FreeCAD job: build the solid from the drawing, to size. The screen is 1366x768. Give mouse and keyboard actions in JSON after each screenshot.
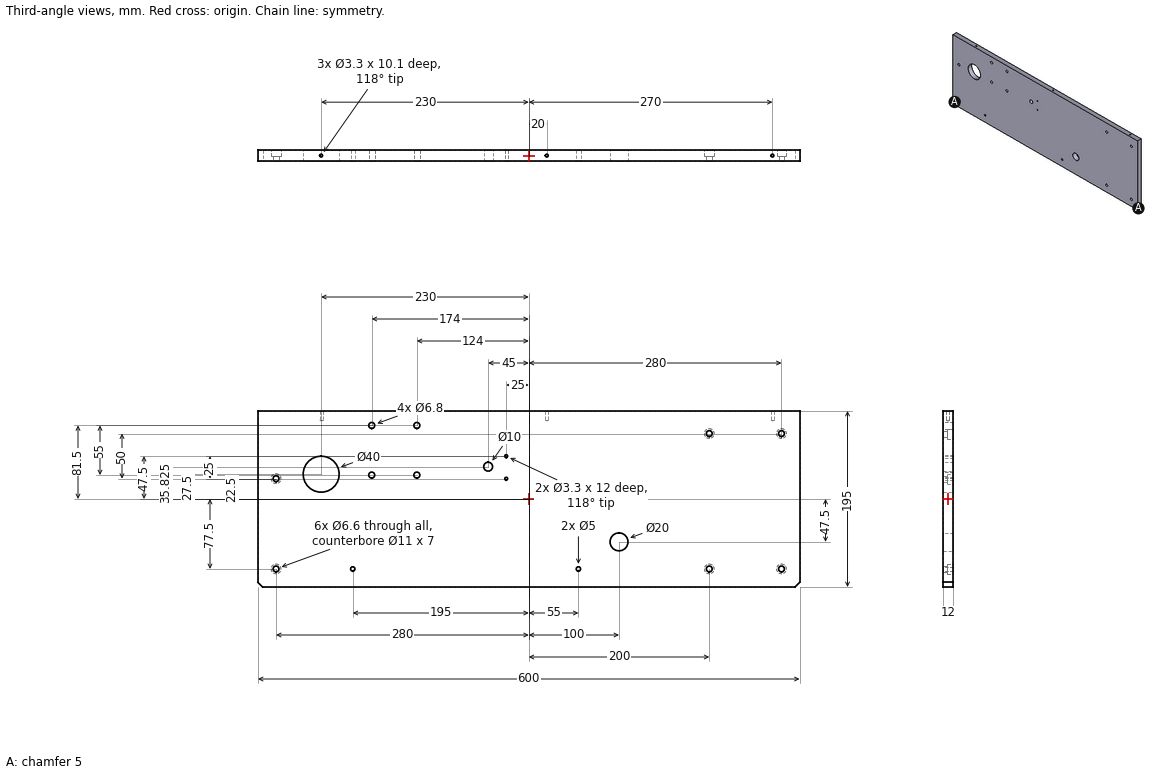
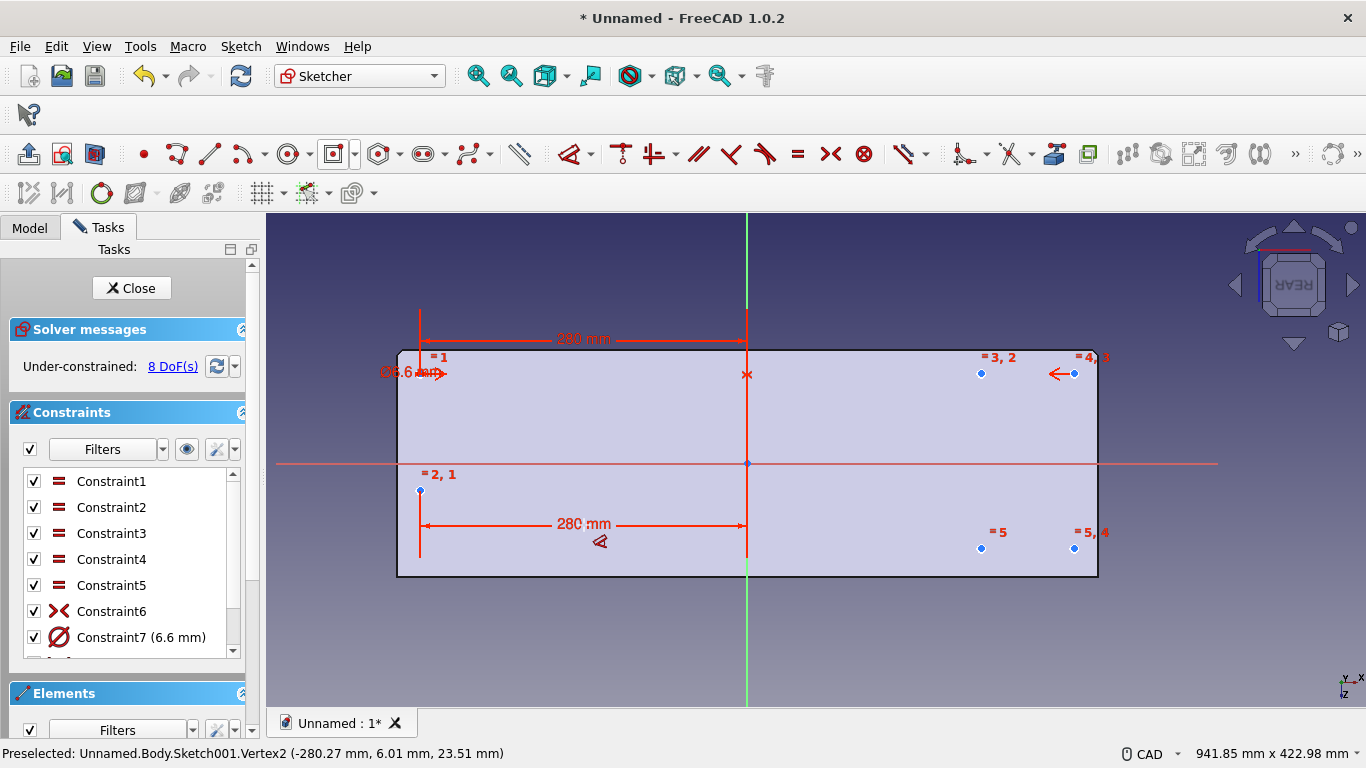
{"action": "left_click", "coordinate": [981, 374]}
{"action": "left_click", "coordinate": [864, 340]}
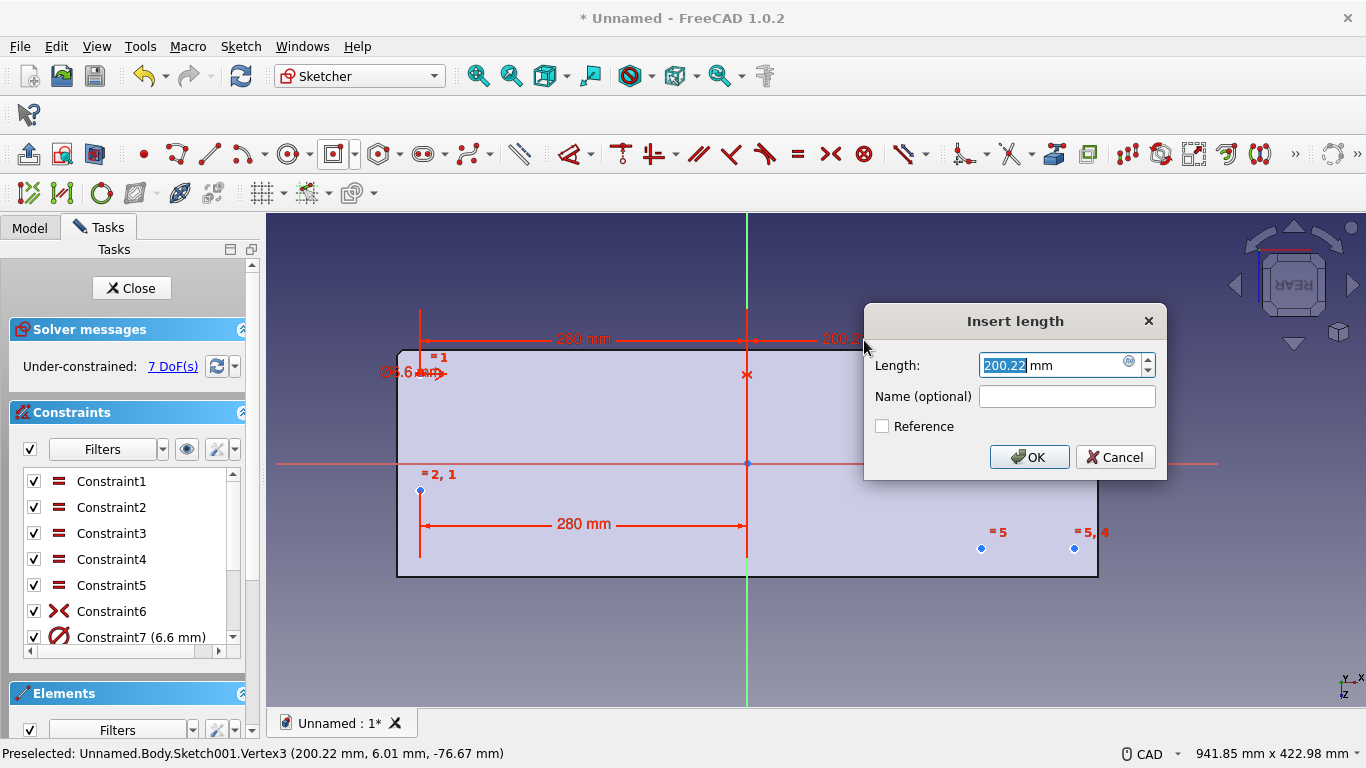
{"action": "type", "text": "200"}
{"action": "key", "text": "Return"}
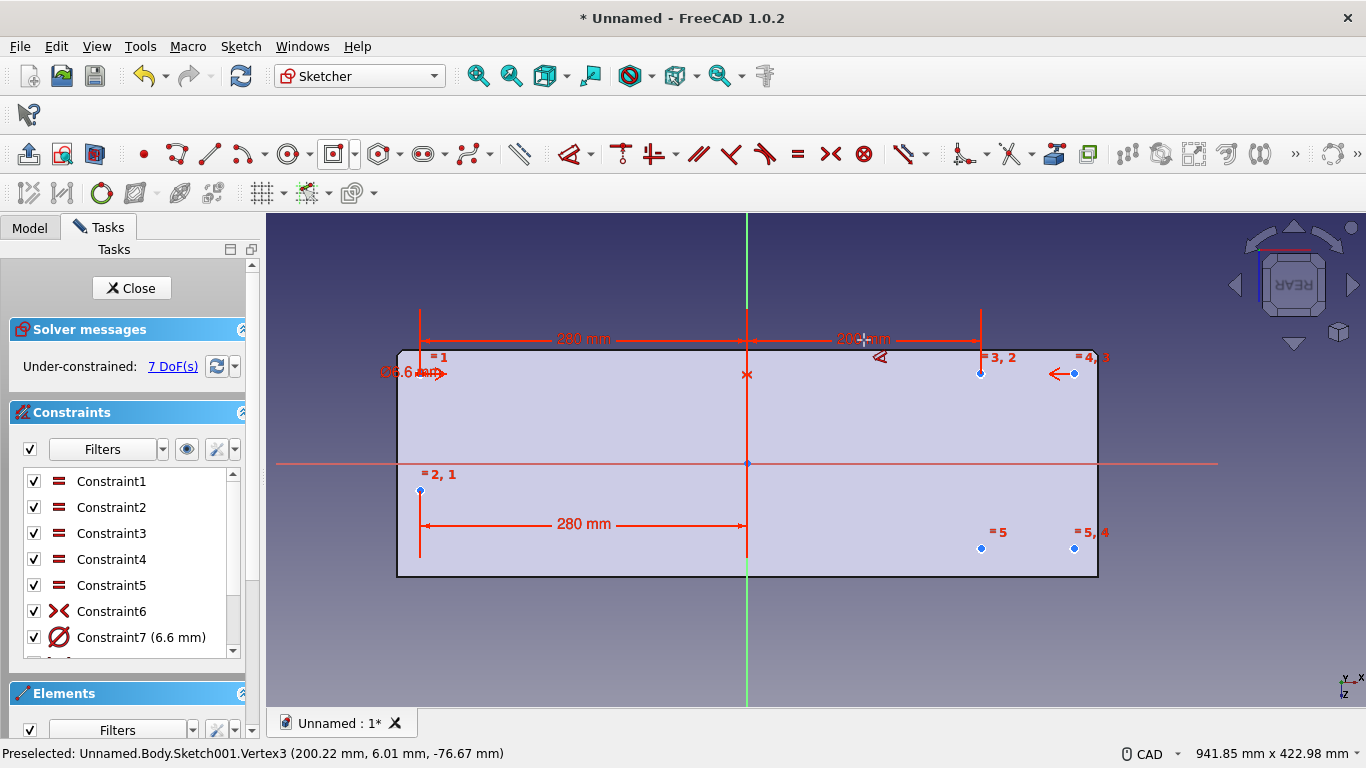
{"action": "left_click", "coordinate": [1074, 549]}
{"action": "left_click", "coordinate": [911, 583]}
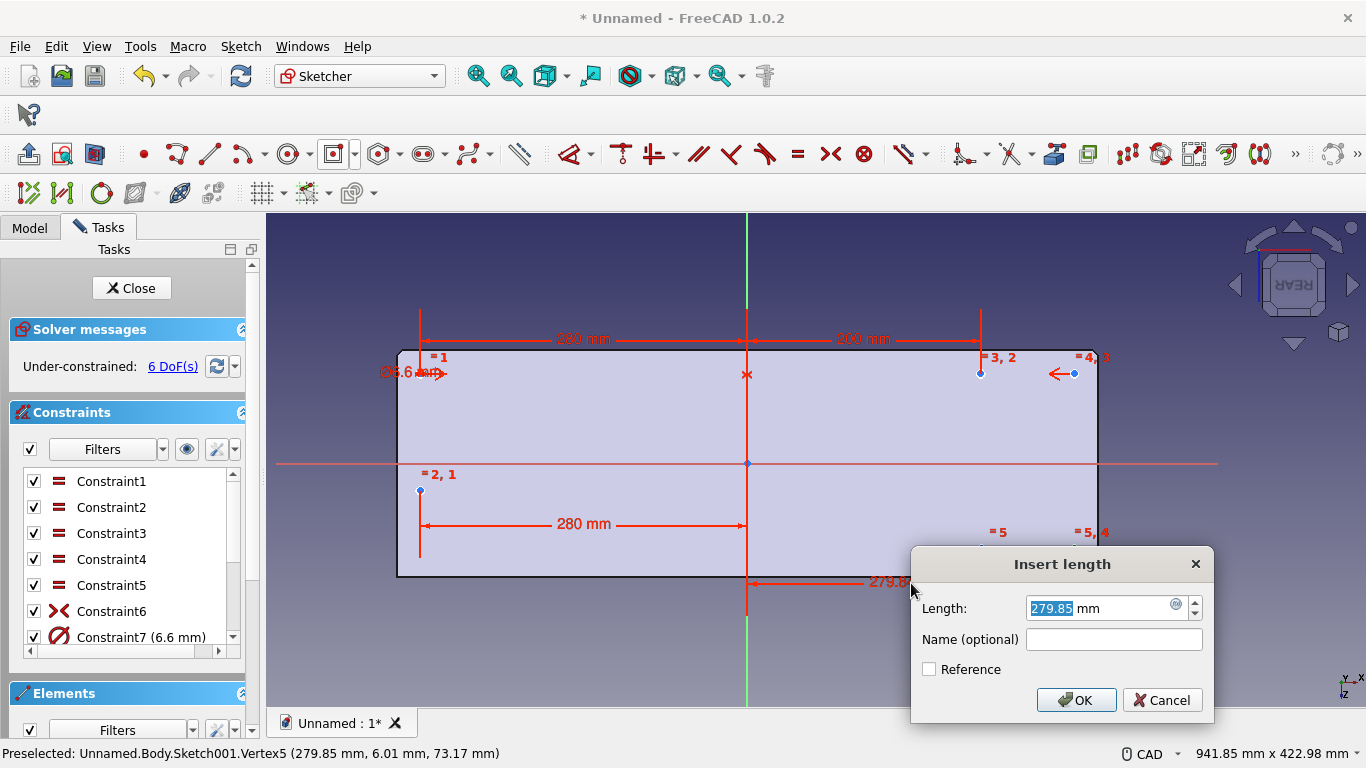
{"action": "type", "text": "280"}
{"action": "key", "text": "Return"}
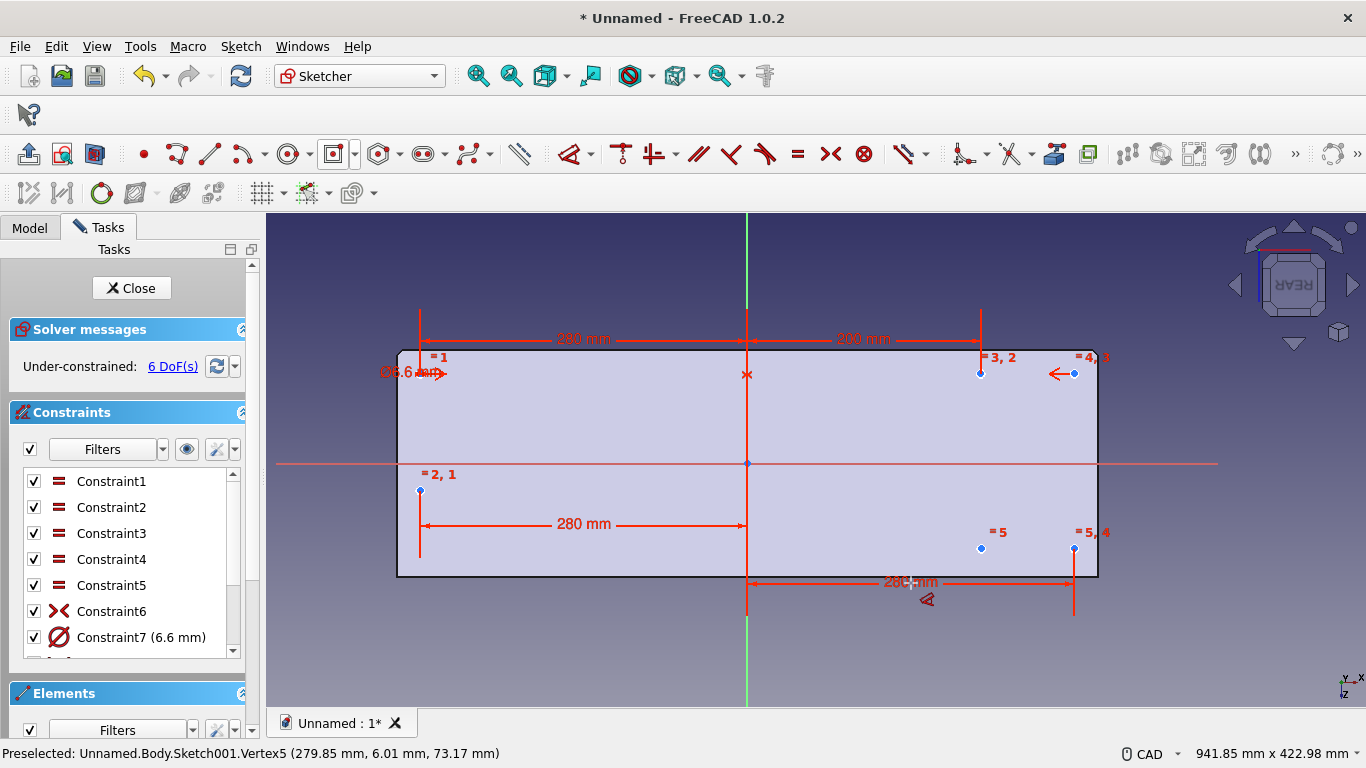
{"action": "left_click", "coordinate": [981, 549]}
{"action": "left_click", "coordinate": [810, 583]}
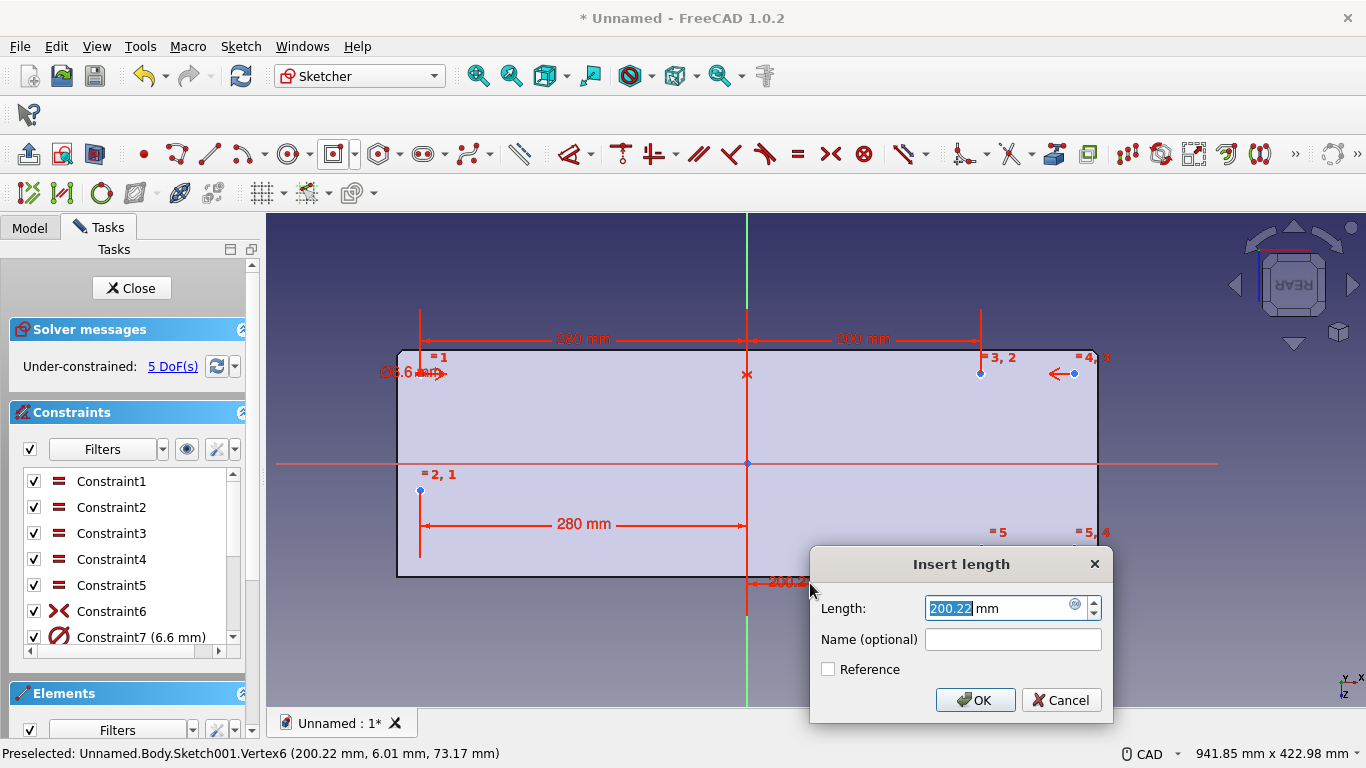
{"action": "type", "text": "200"}
{"action": "key", "text": "Return"}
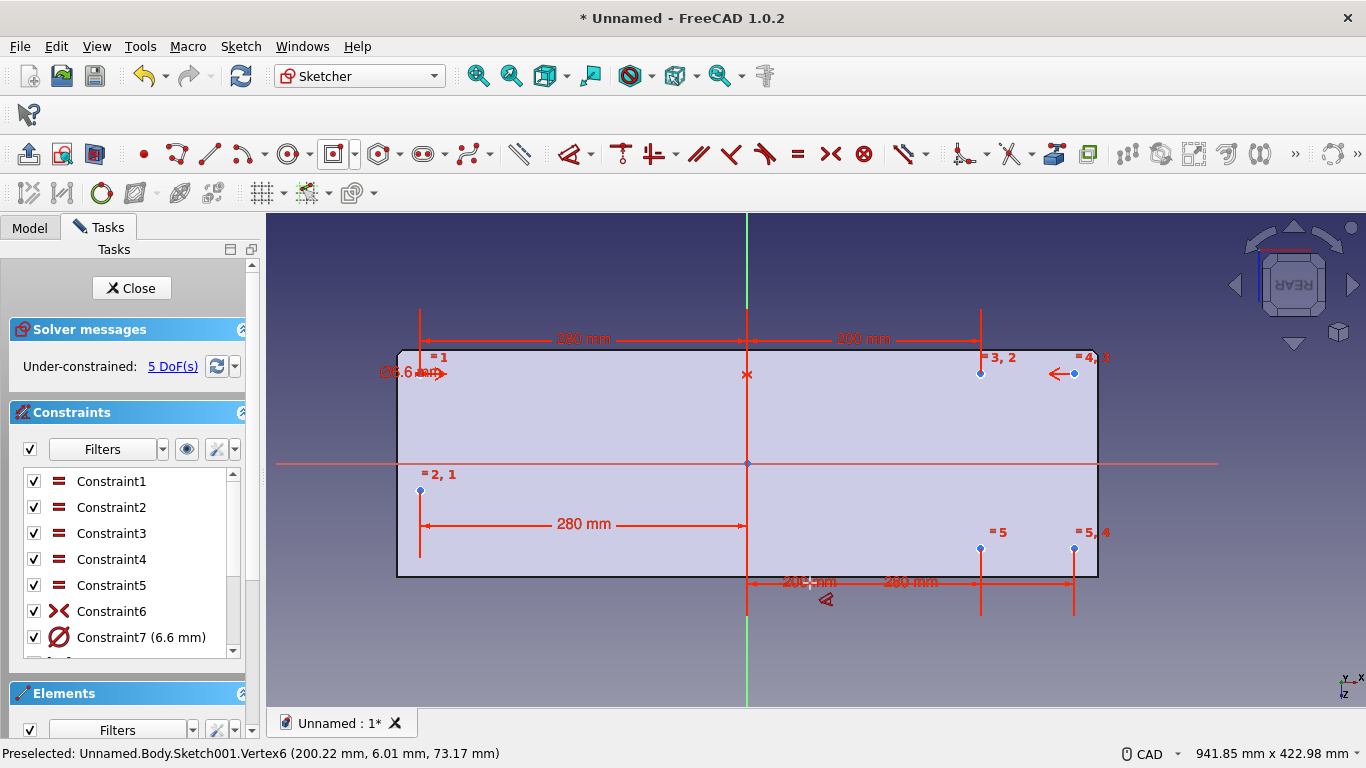
{"action": "left_click", "coordinate": [420, 491]}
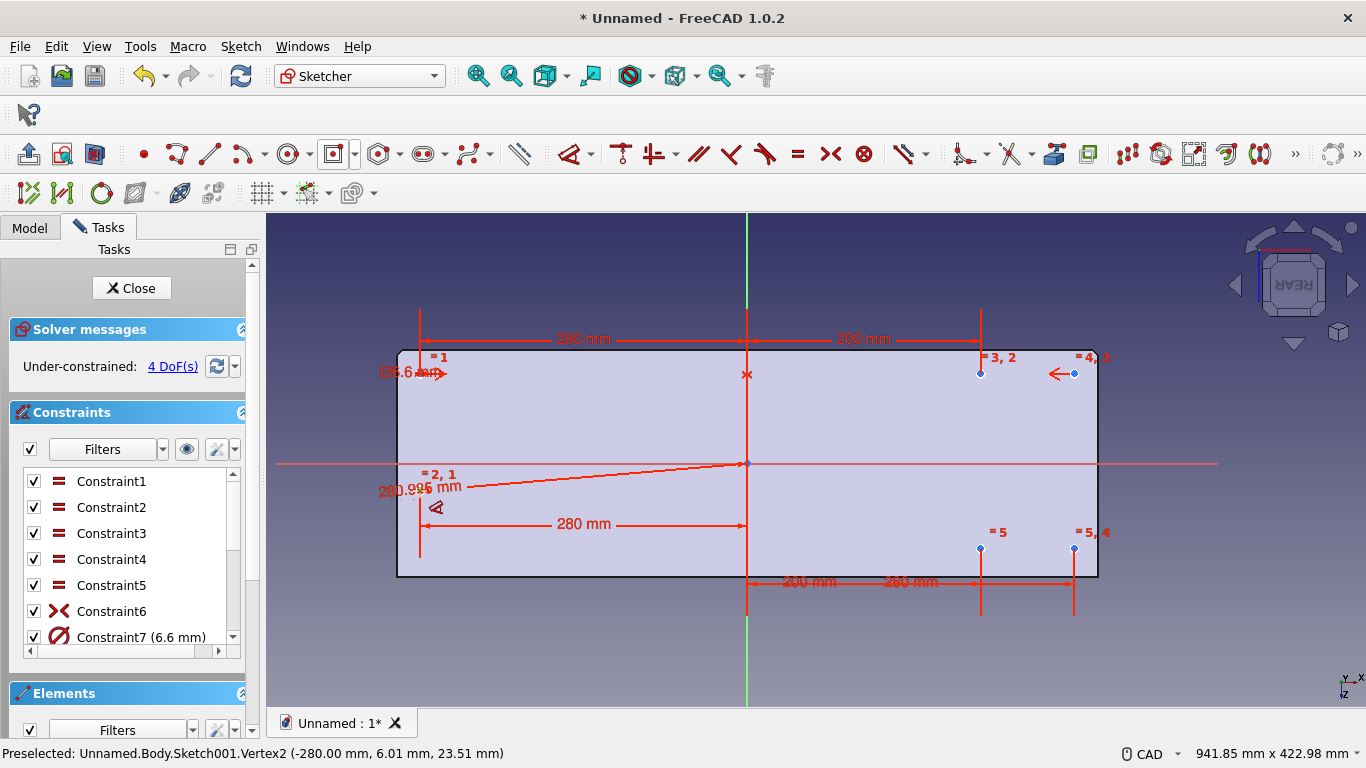
{"action": "left_click", "coordinate": [1074, 549]}
{"action": "left_click", "coordinate": [1108, 520]}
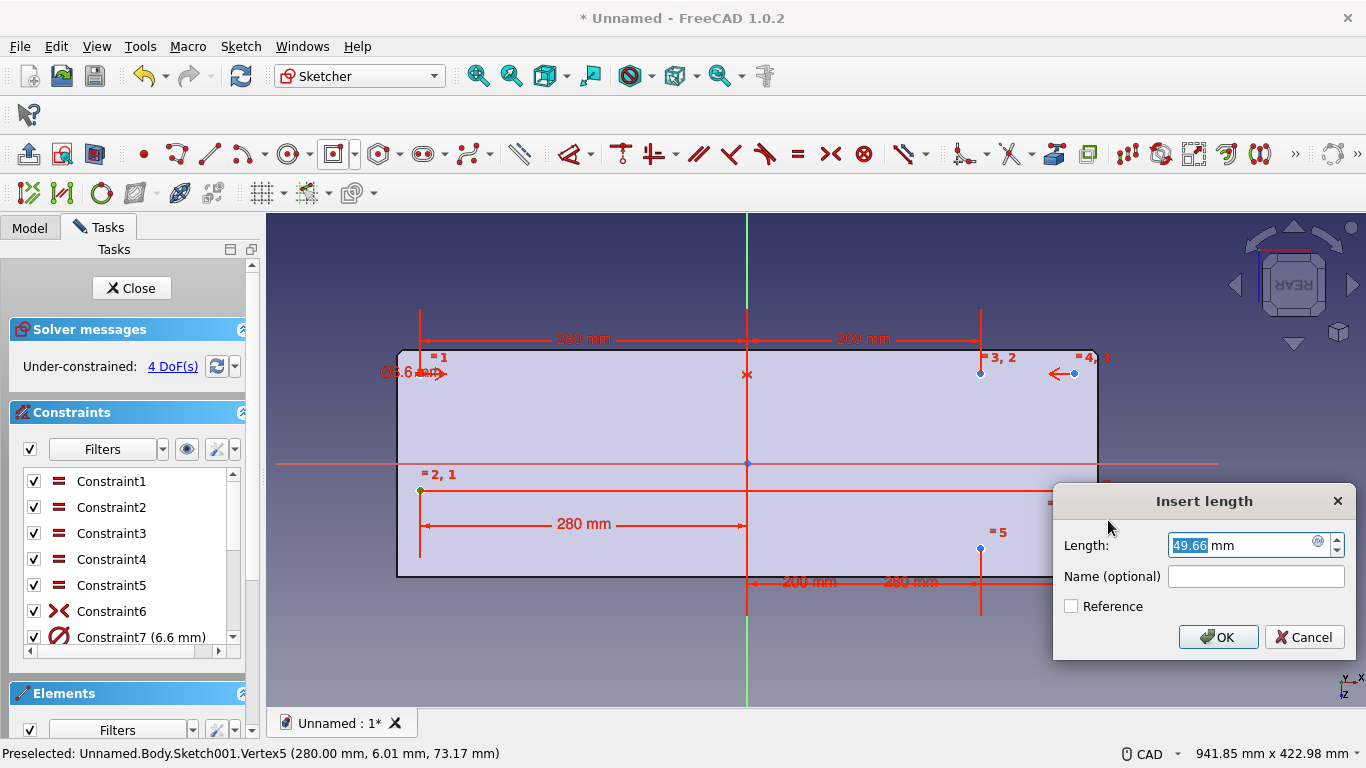
{"action": "type", "text": "50"}
{"action": "key", "text": "Return"}